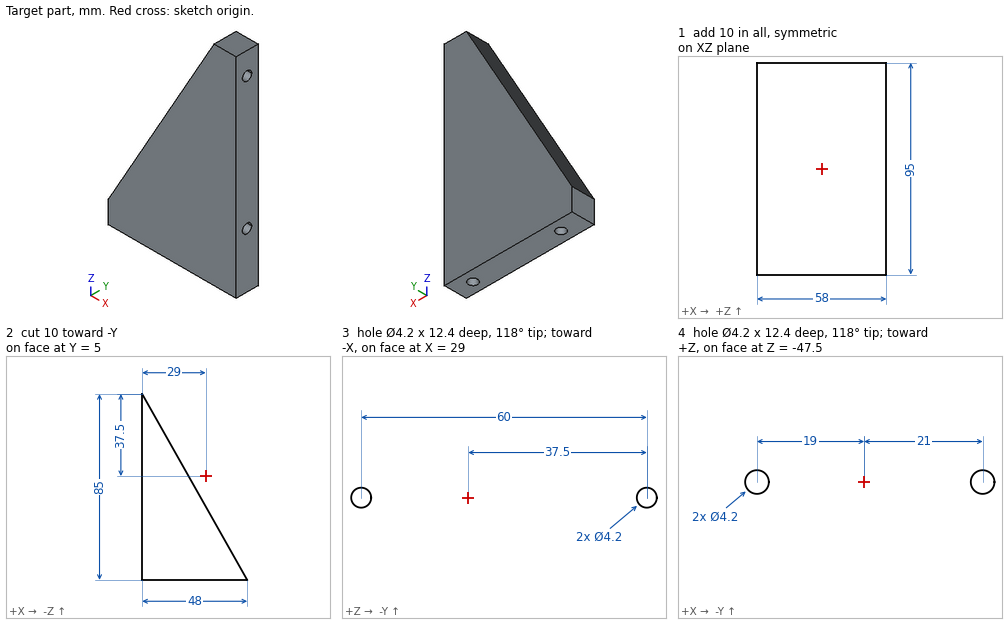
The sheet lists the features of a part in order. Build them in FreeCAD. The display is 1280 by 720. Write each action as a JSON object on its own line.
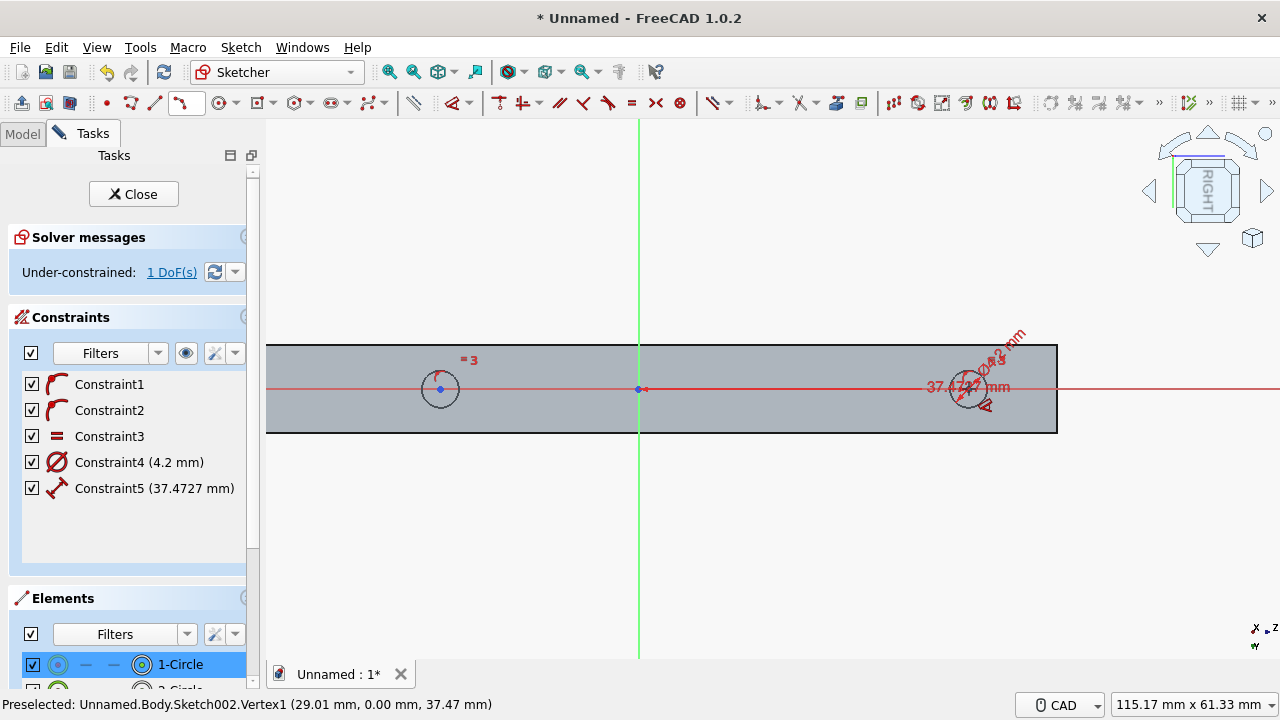
{"action": "left_click", "coordinate": [440, 389]}
{"action": "left_click", "coordinate": [704, 423]}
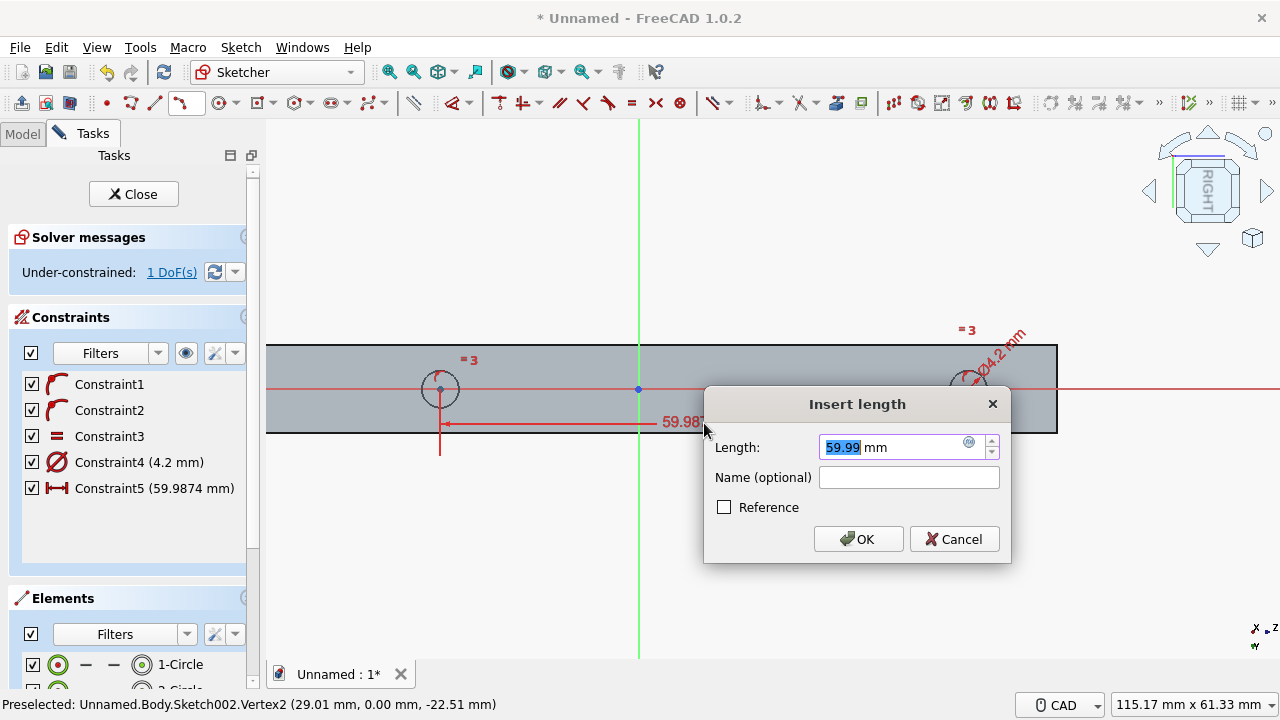
{"action": "type", "text": "60"}
{"action": "key", "text": "Return"}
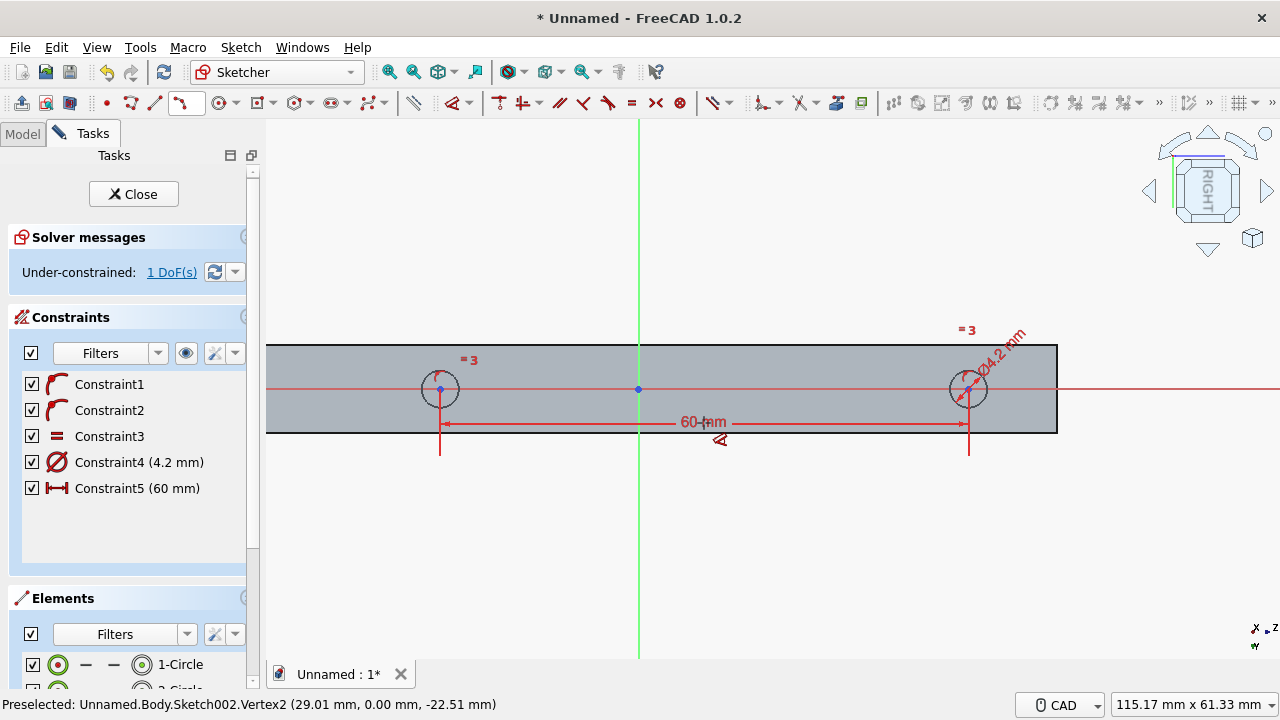
{"action": "left_click", "coordinate": [969, 389]}
{"action": "left_click", "coordinate": [804, 423]}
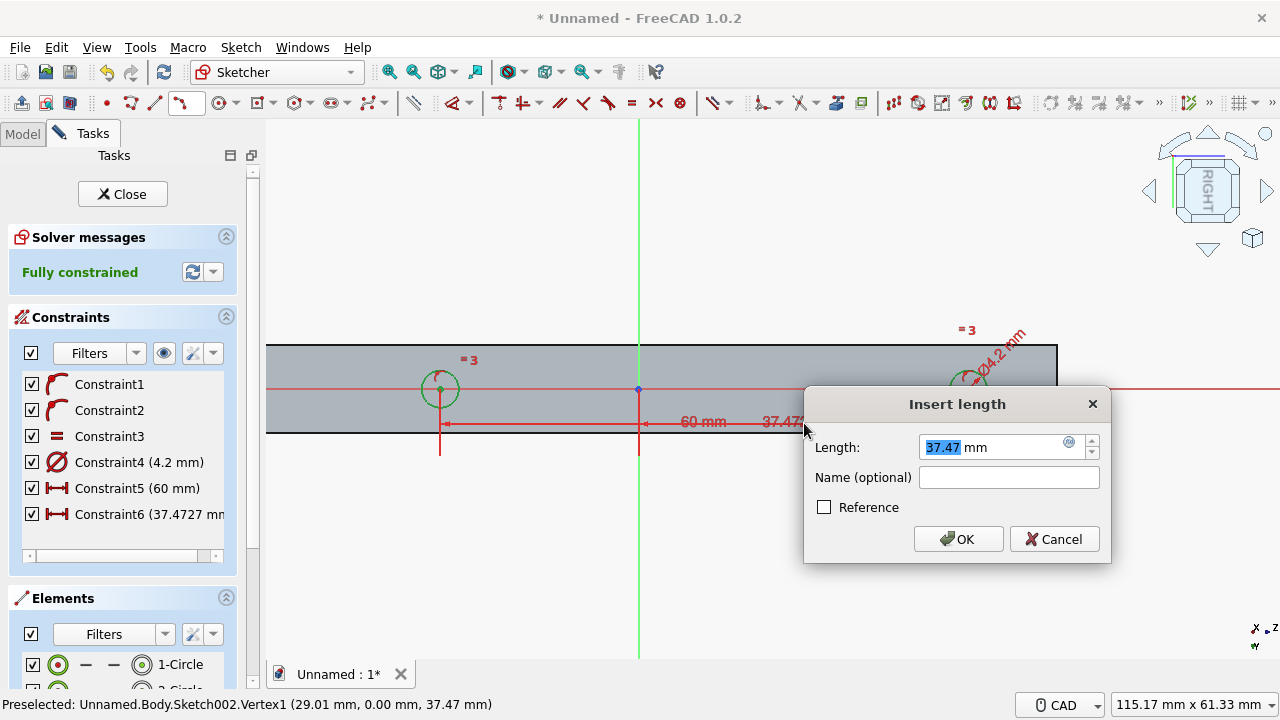
{"action": "type", "text": "37.5"}
{"action": "key", "text": "Return"}
{"action": "key", "text": "Escape"}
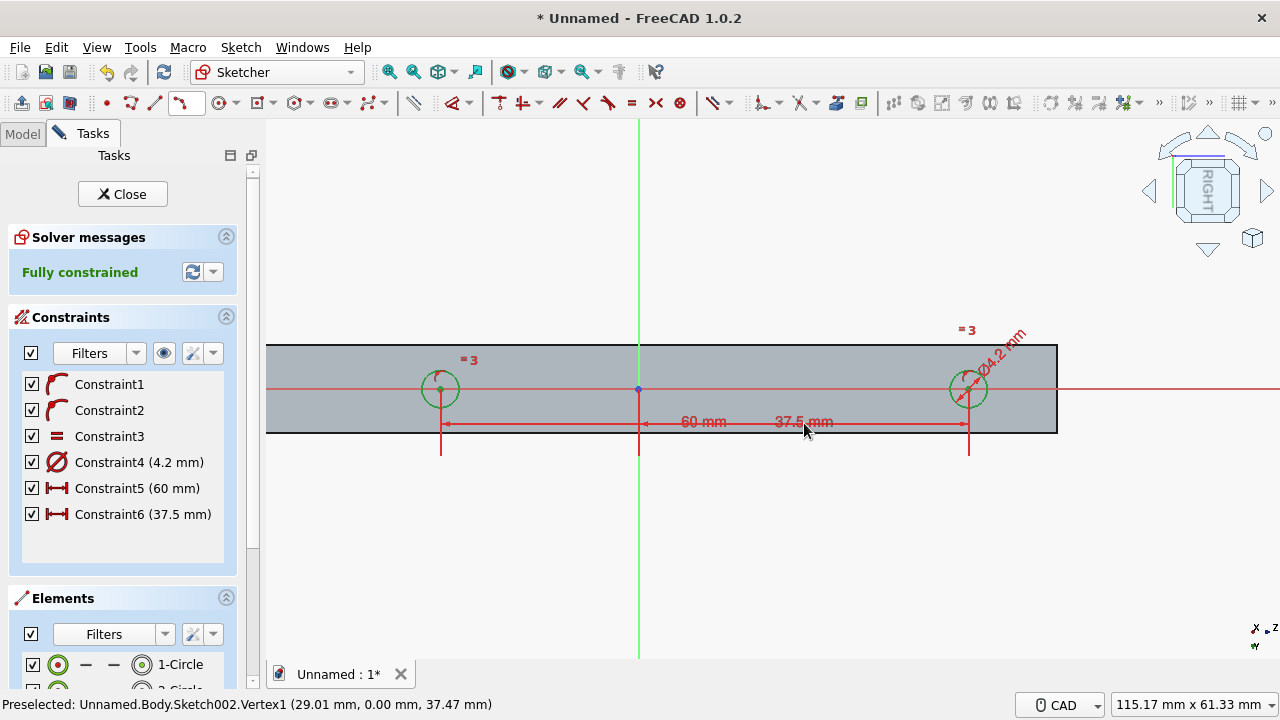
{"action": "left_click", "coordinate": [123, 194]}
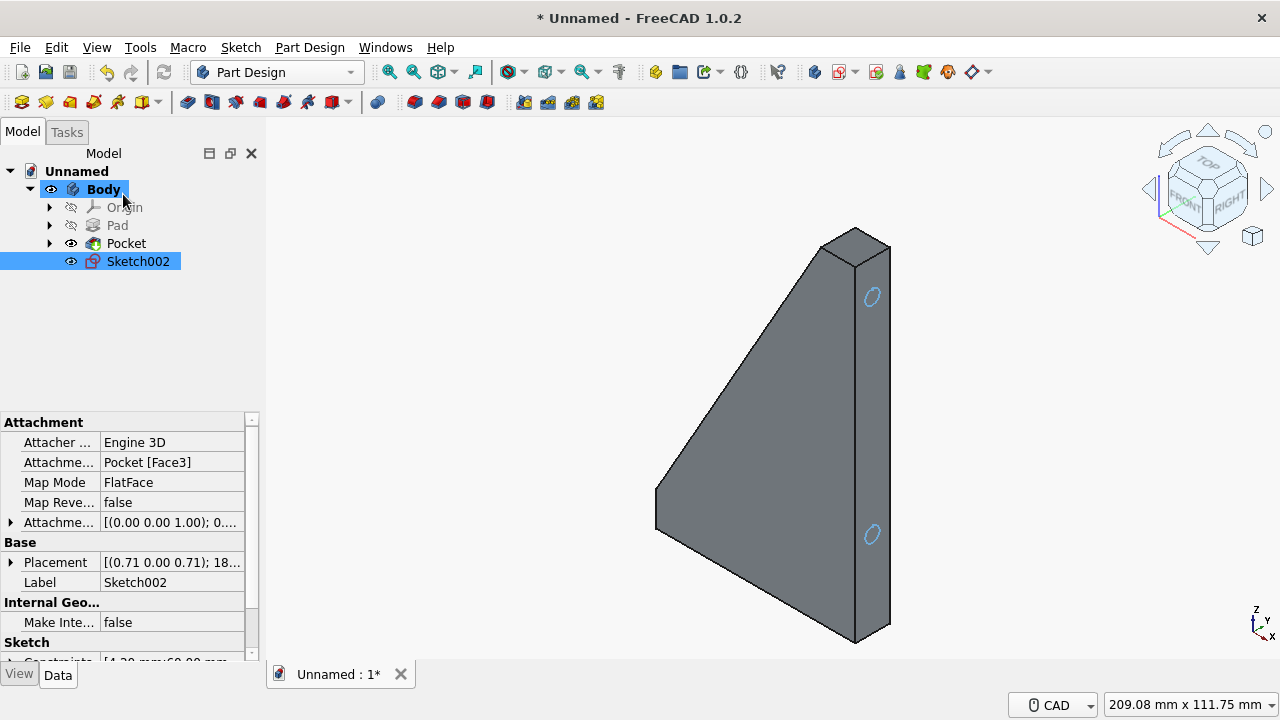
{"action": "left_click", "coordinate": [212, 102]}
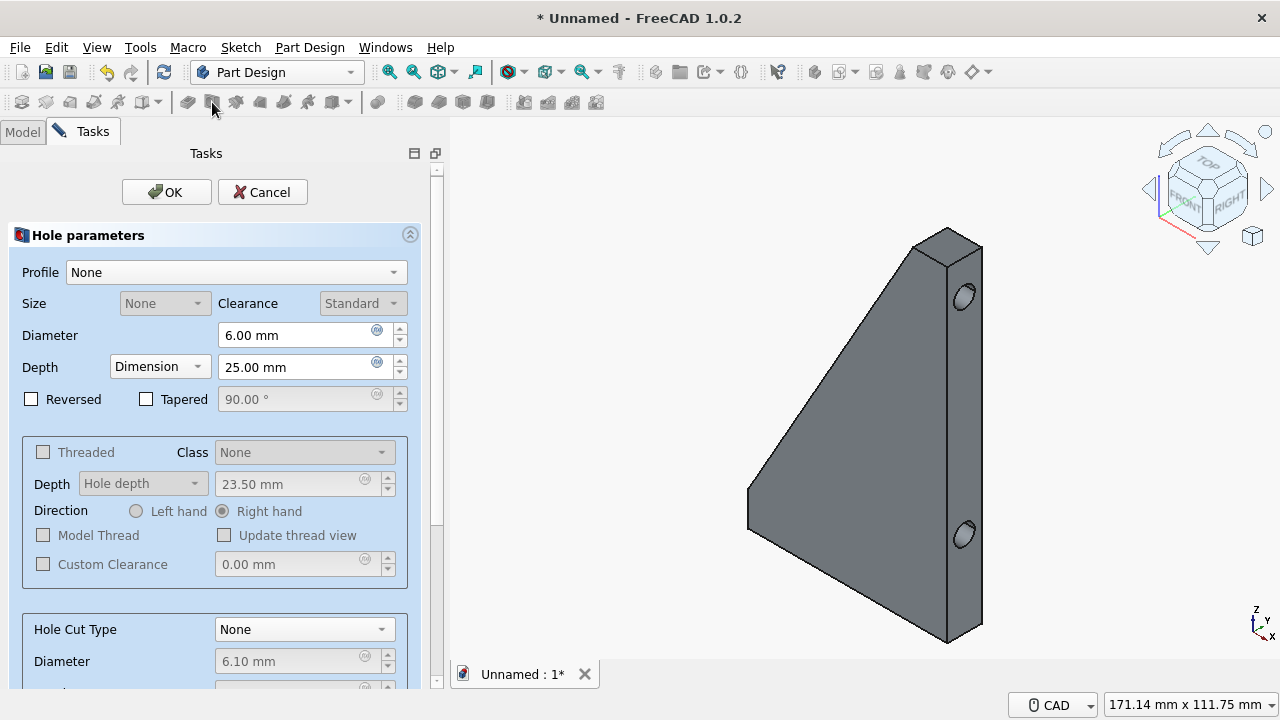
{"action": "triple_click", "coordinate": [305, 335]}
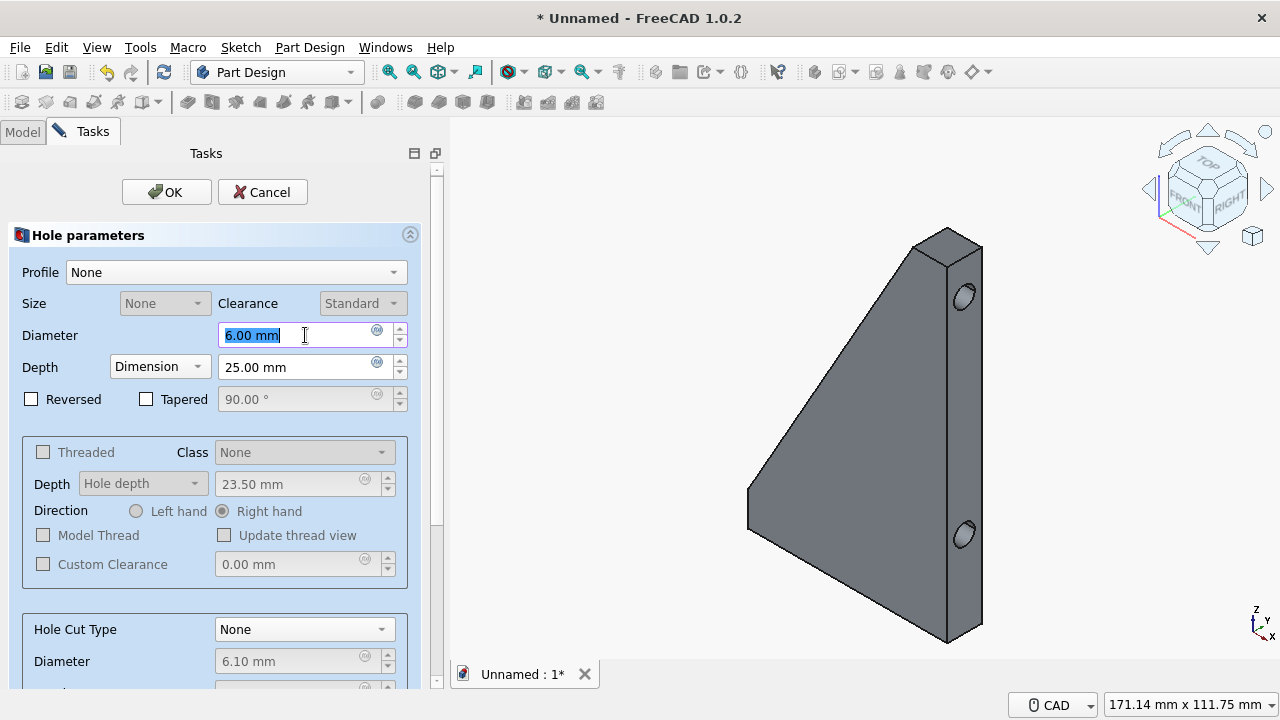
{"action": "type", "text": "4.2"}
{"action": "key", "text": "Tab"}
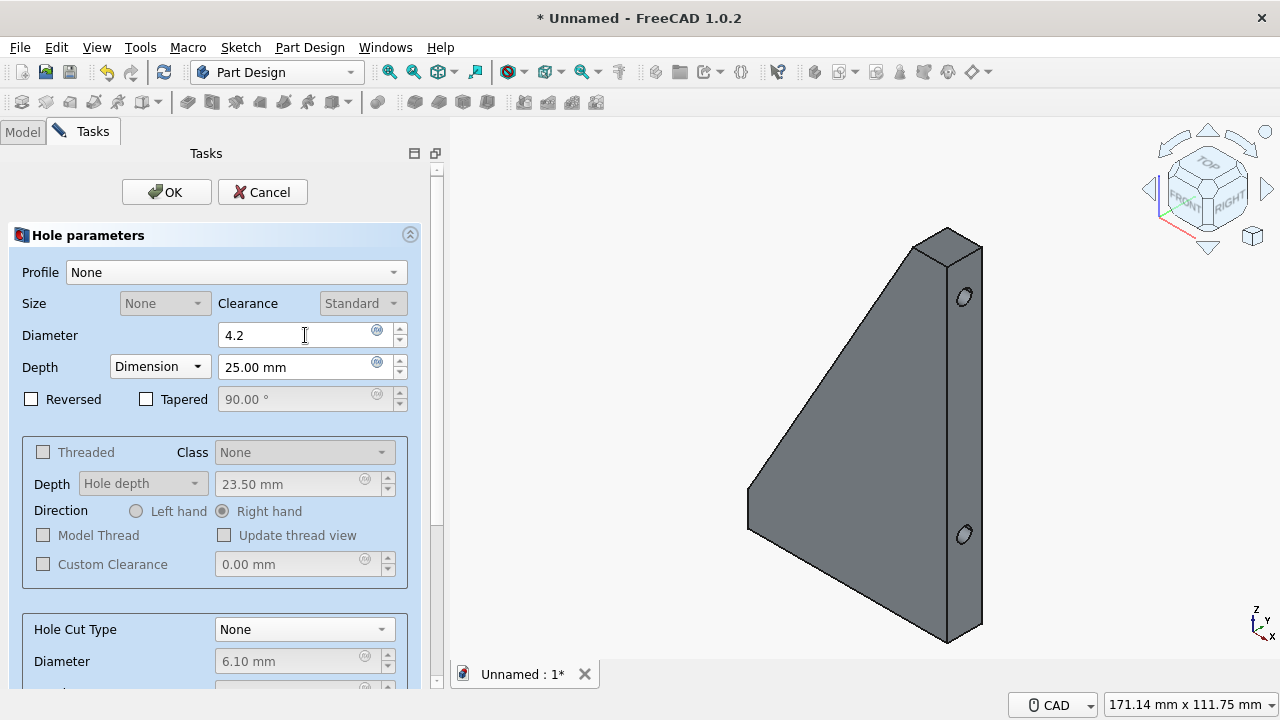
{"action": "triple_click", "coordinate": [305, 367]}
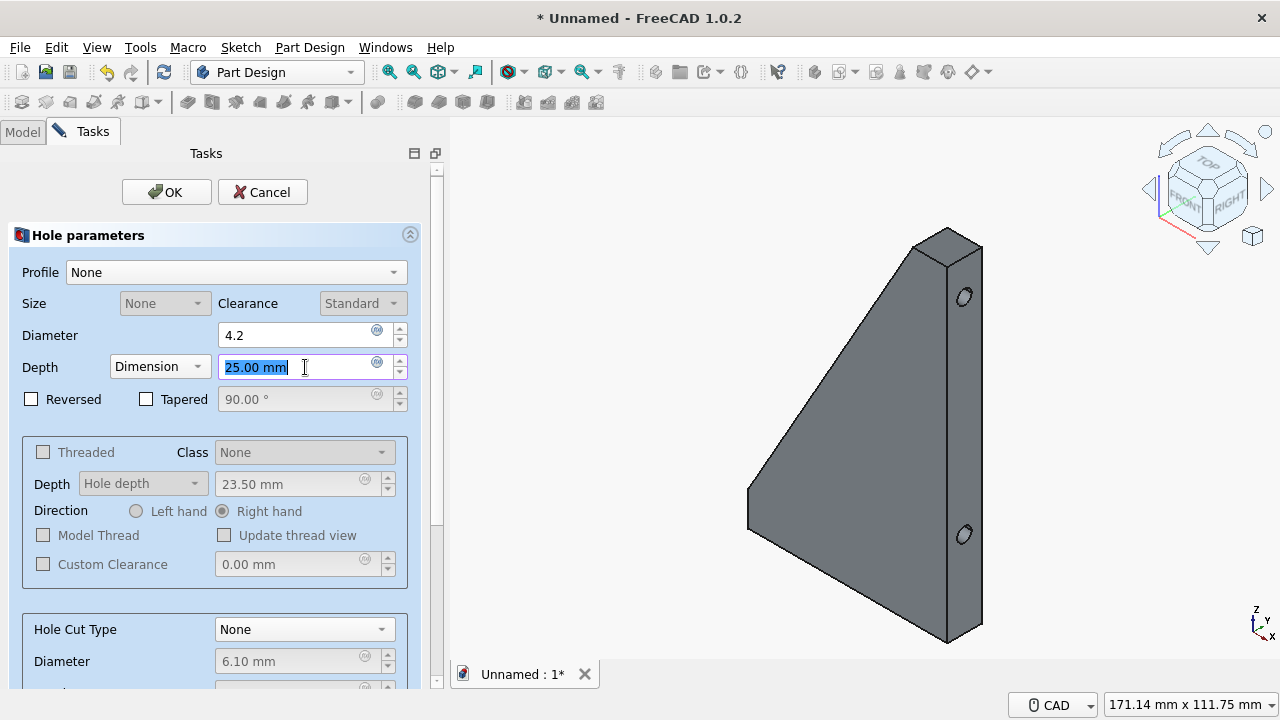
{"action": "type", "text": "12.4"}
{"action": "key", "text": "Tab"}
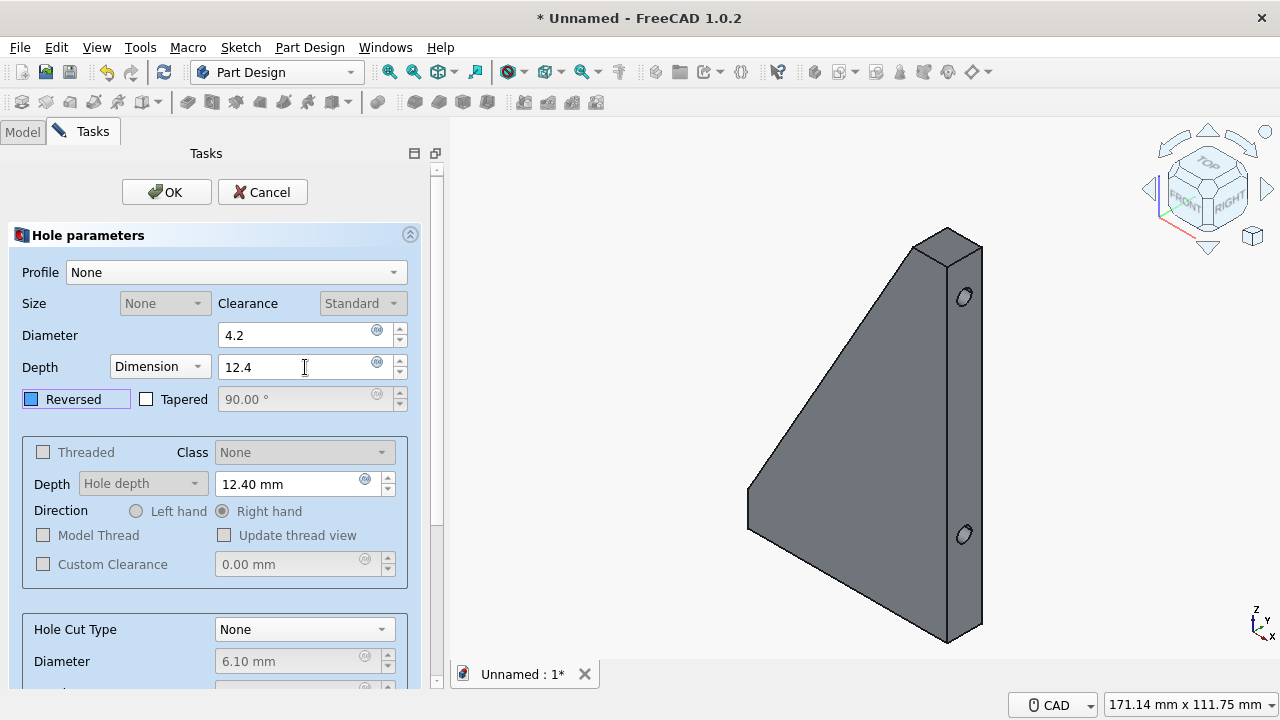
{"action": "left_click", "coordinate": [167, 192]}